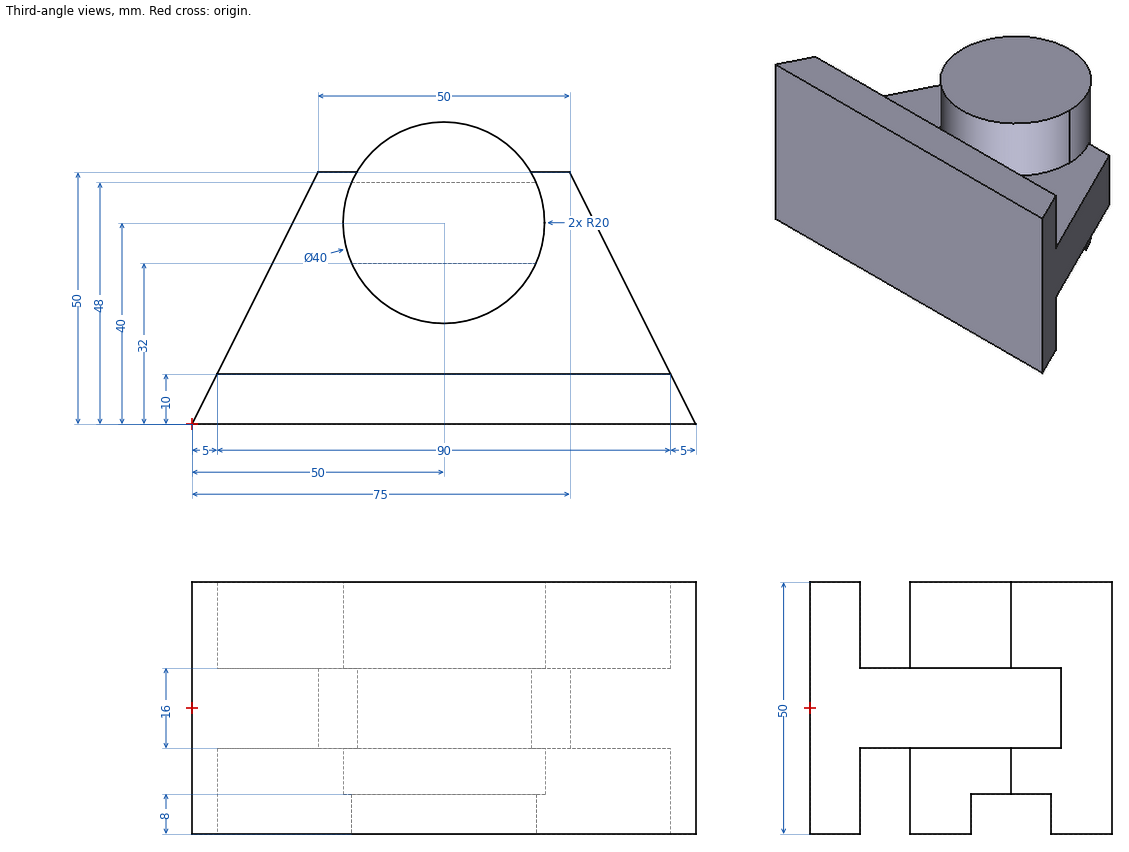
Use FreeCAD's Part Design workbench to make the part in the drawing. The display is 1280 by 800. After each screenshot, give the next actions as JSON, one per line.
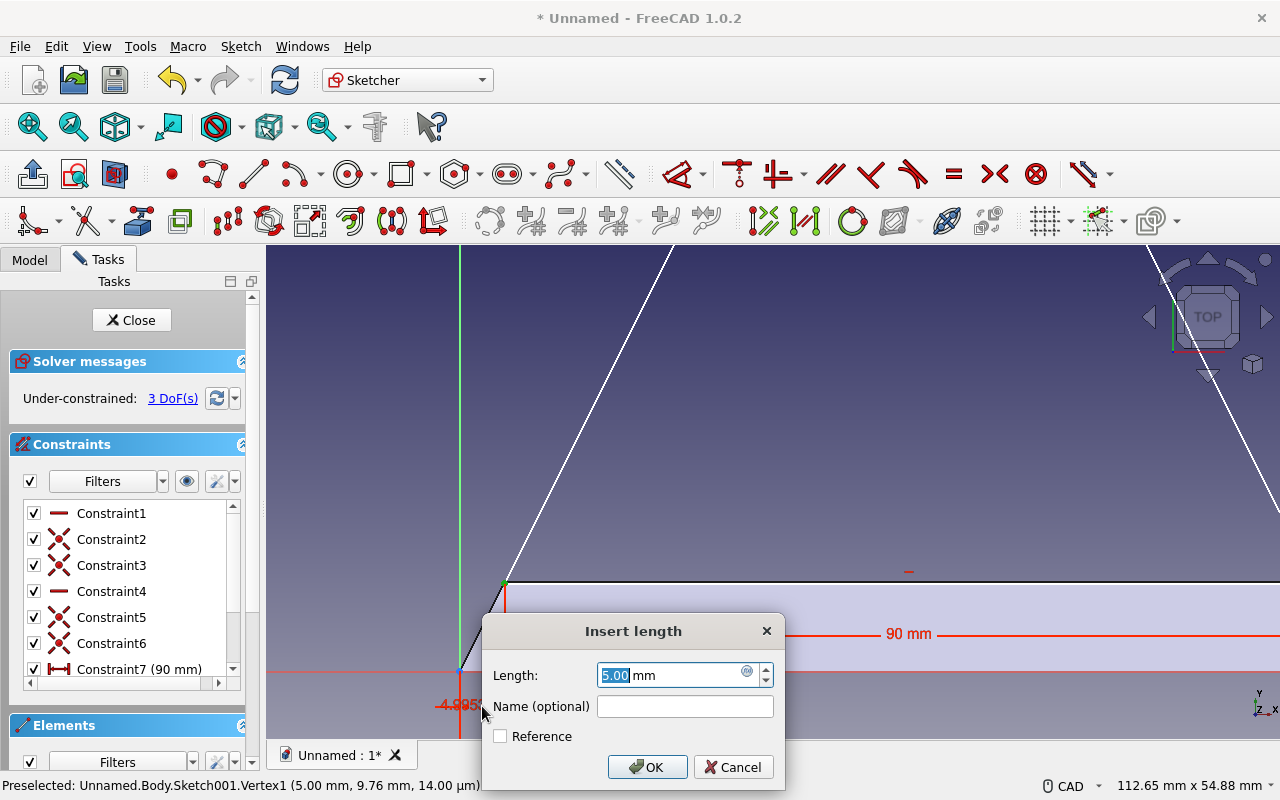
{"action": "type", "text": "5"}
{"action": "key", "text": "Return"}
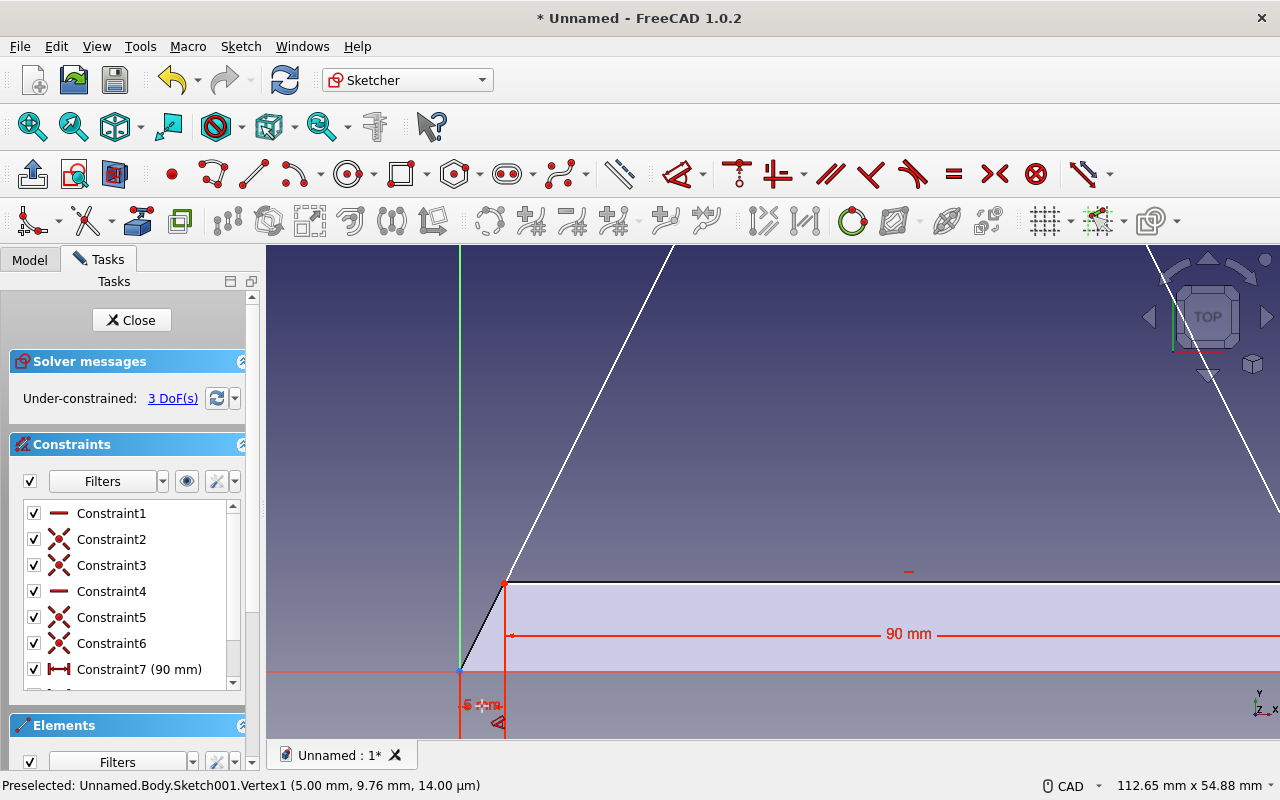
{"action": "left_click", "coordinate": [505, 584]}
{"action": "left_click", "coordinate": [426, 628]}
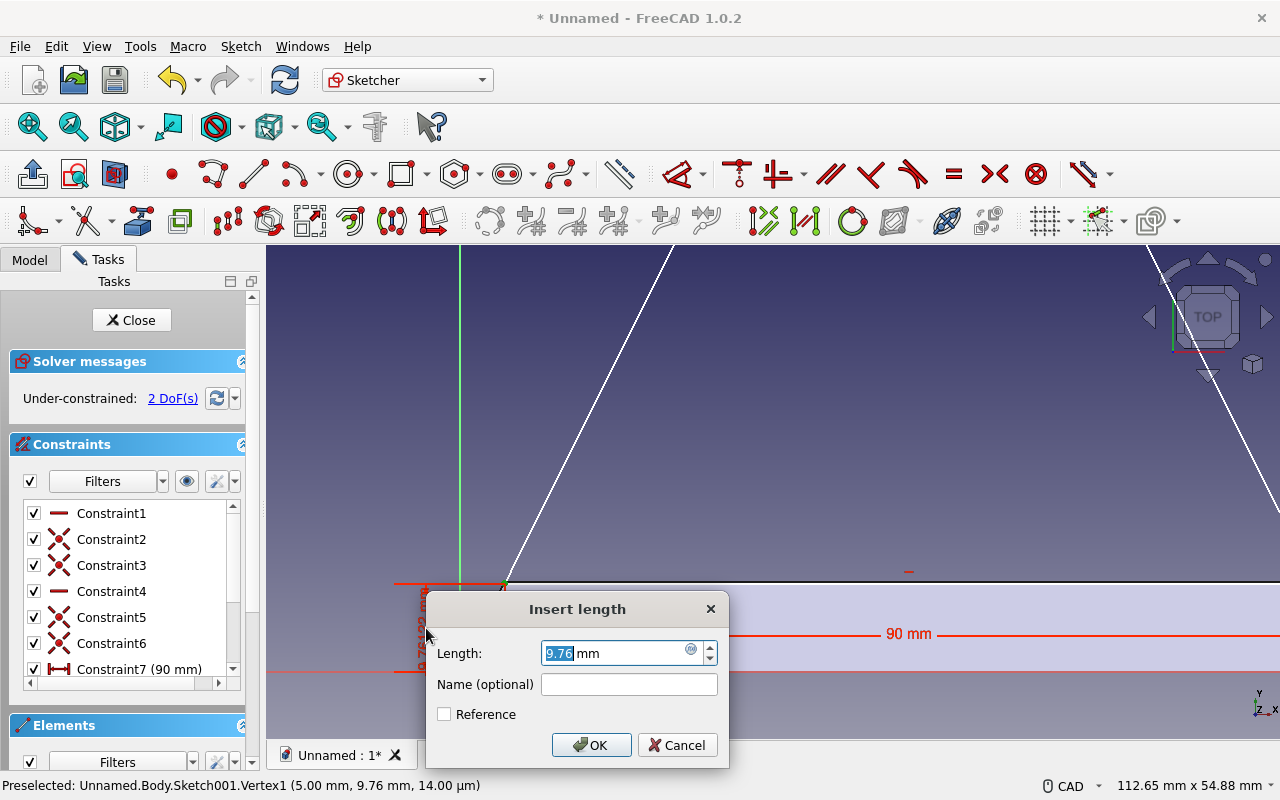
{"action": "type", "text": "10"}
{"action": "key", "text": "Return"}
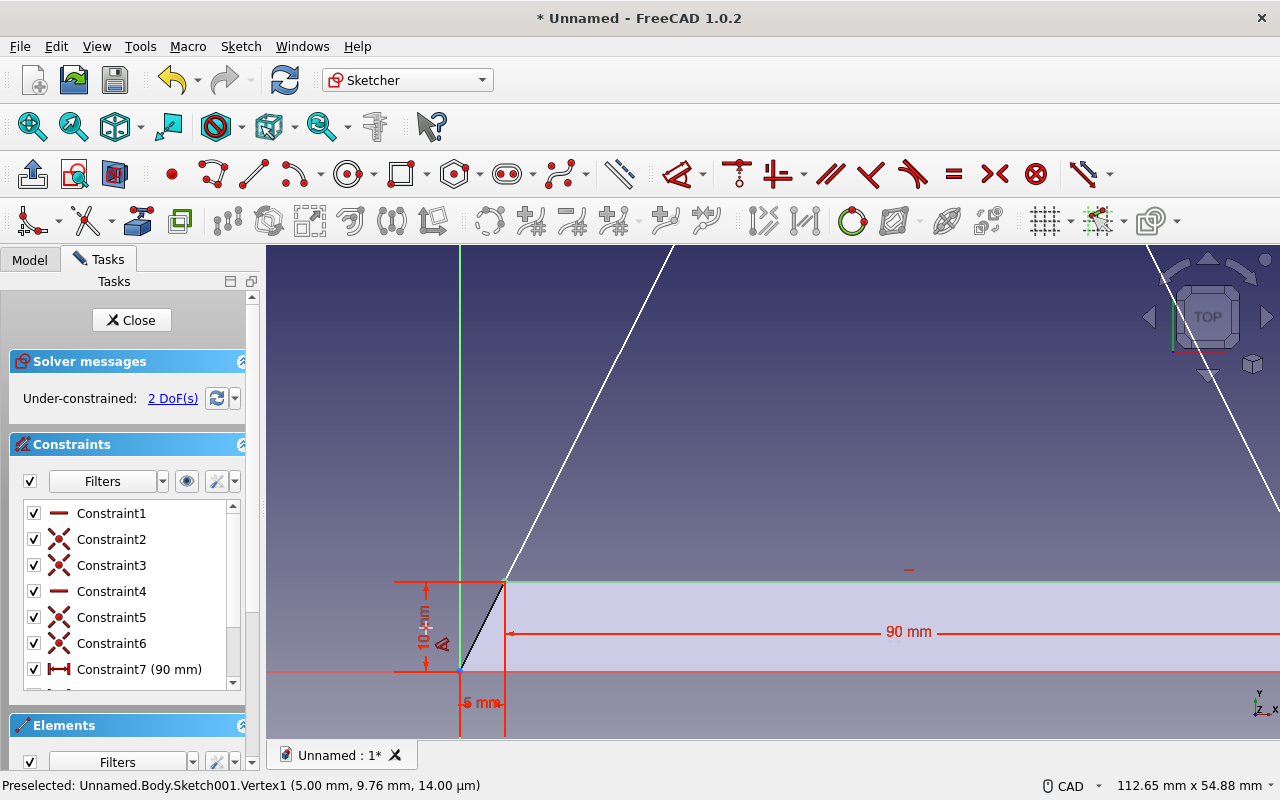
{"action": "scroll", "coordinate": [332, 585], "scroll_direction": "down", "scroll_amount": 2}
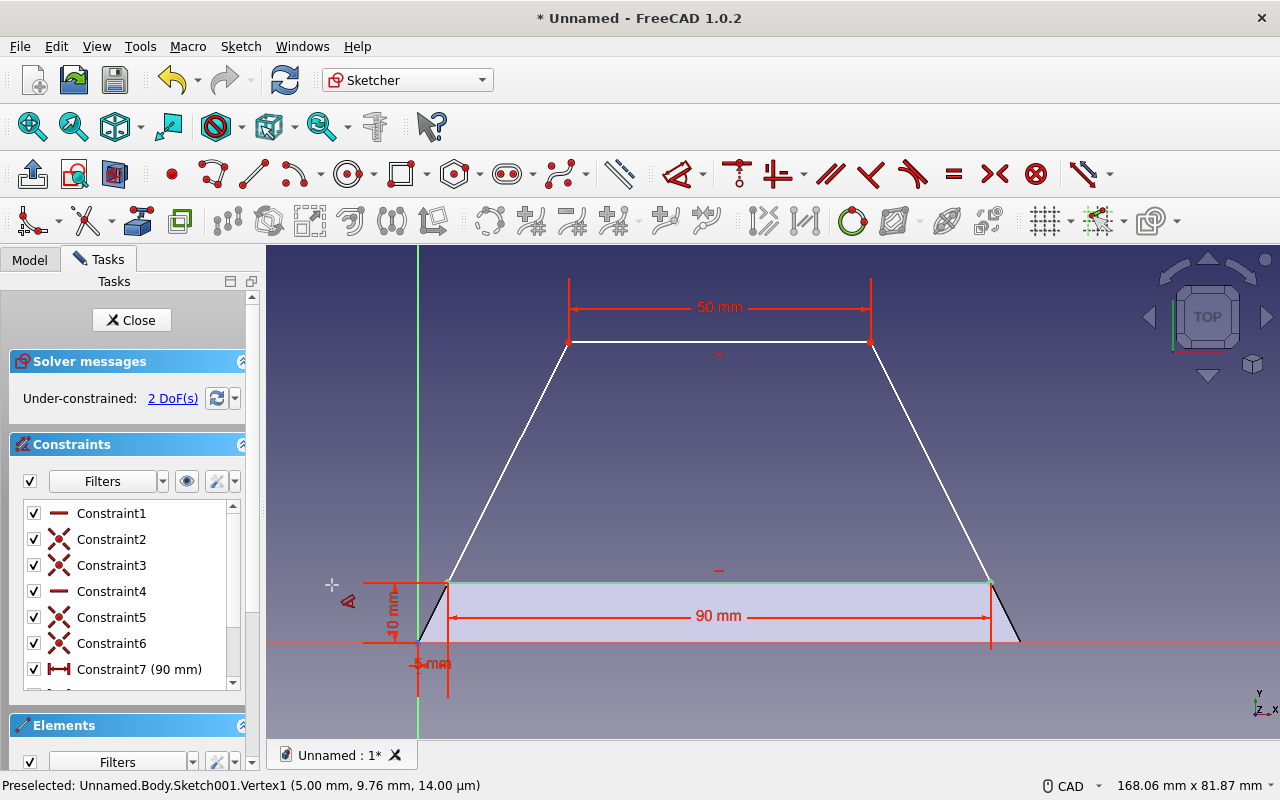
{"action": "left_click", "coordinate": [871, 342]}
{"action": "left_click", "coordinate": [644, 677]}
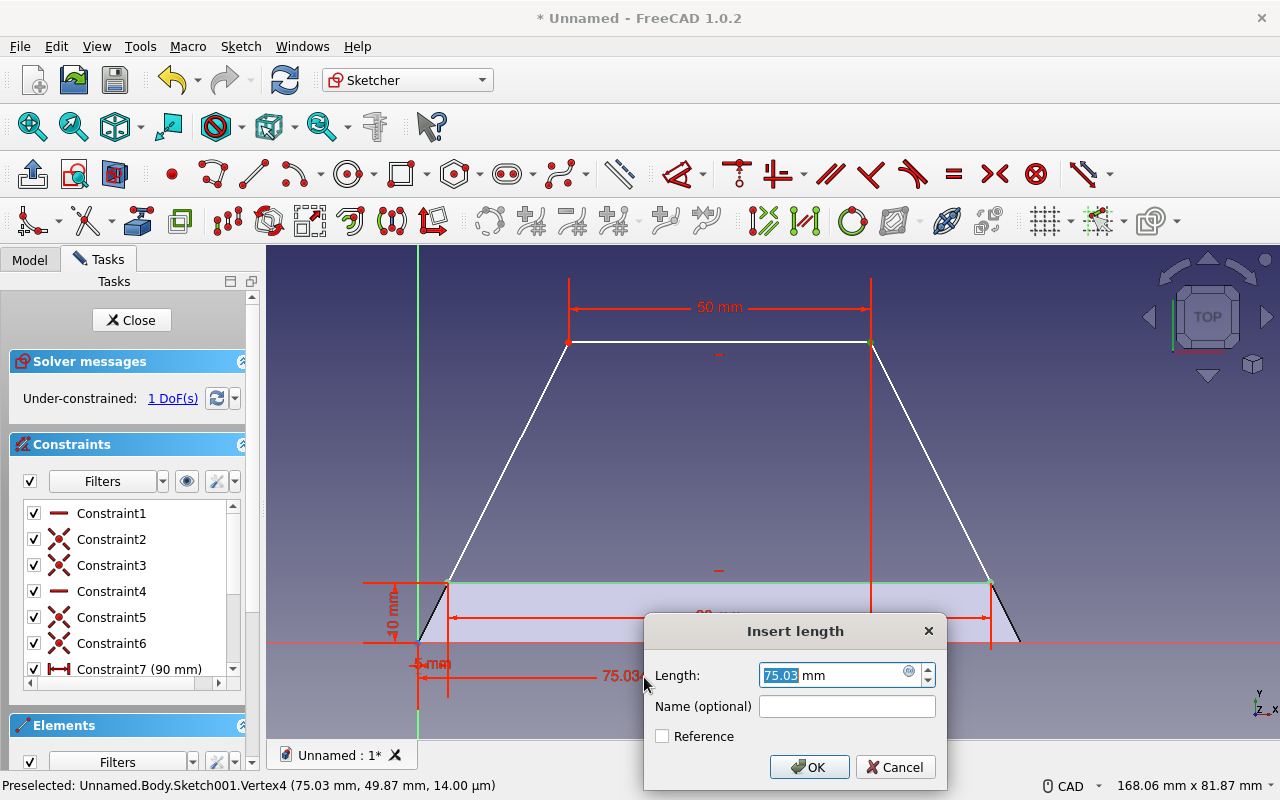
{"action": "type", "text": "75"}
{"action": "key", "text": "Return"}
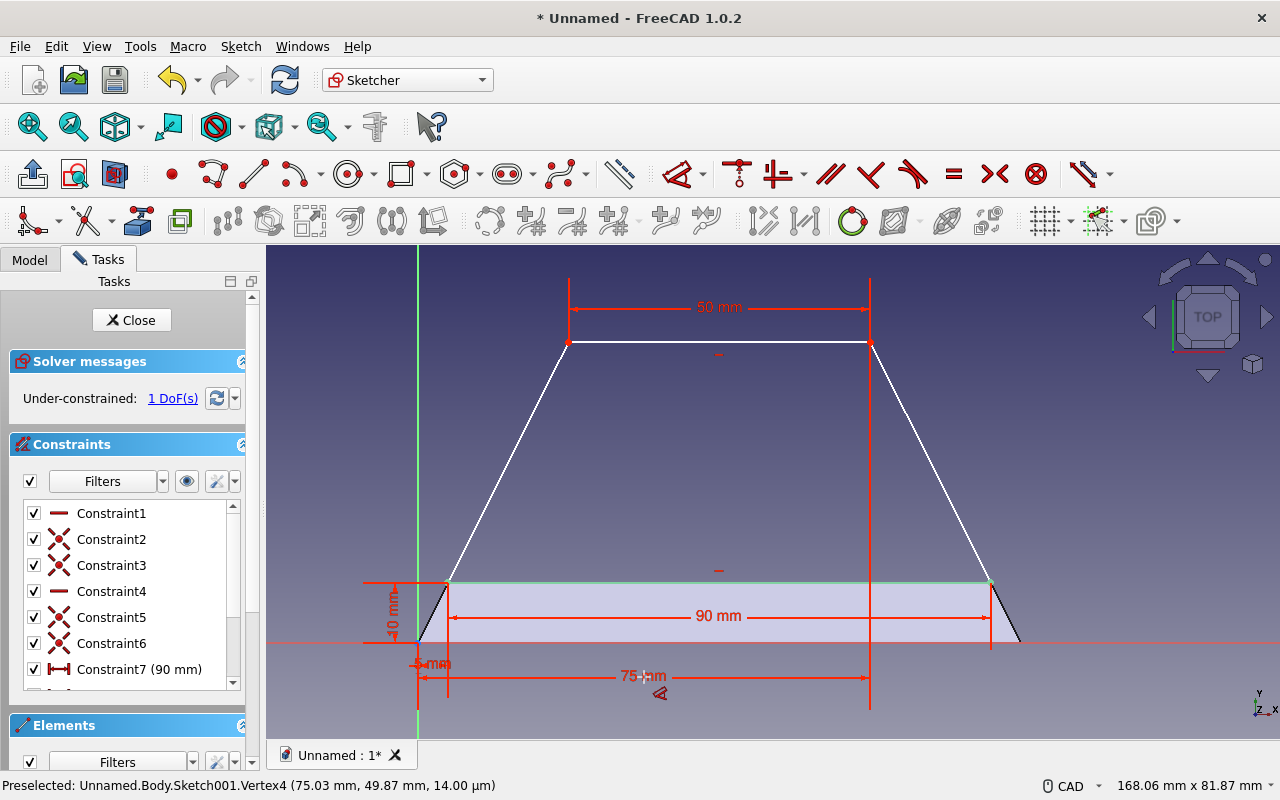
{"action": "left_click", "coordinate": [870, 342]}
{"action": "left_click", "coordinate": [384, 493]}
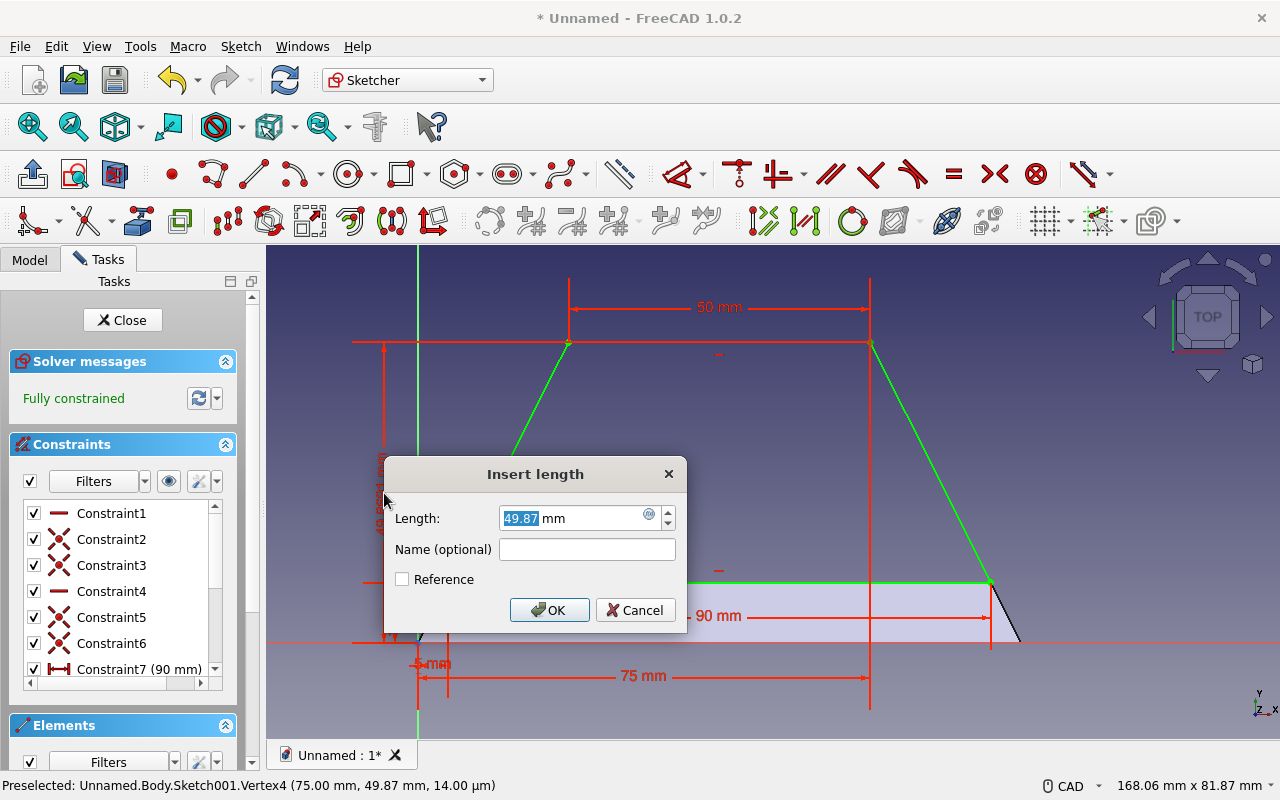
{"action": "type", "text": "50"}
{"action": "key", "text": "Return"}
{"action": "key", "text": "Escape"}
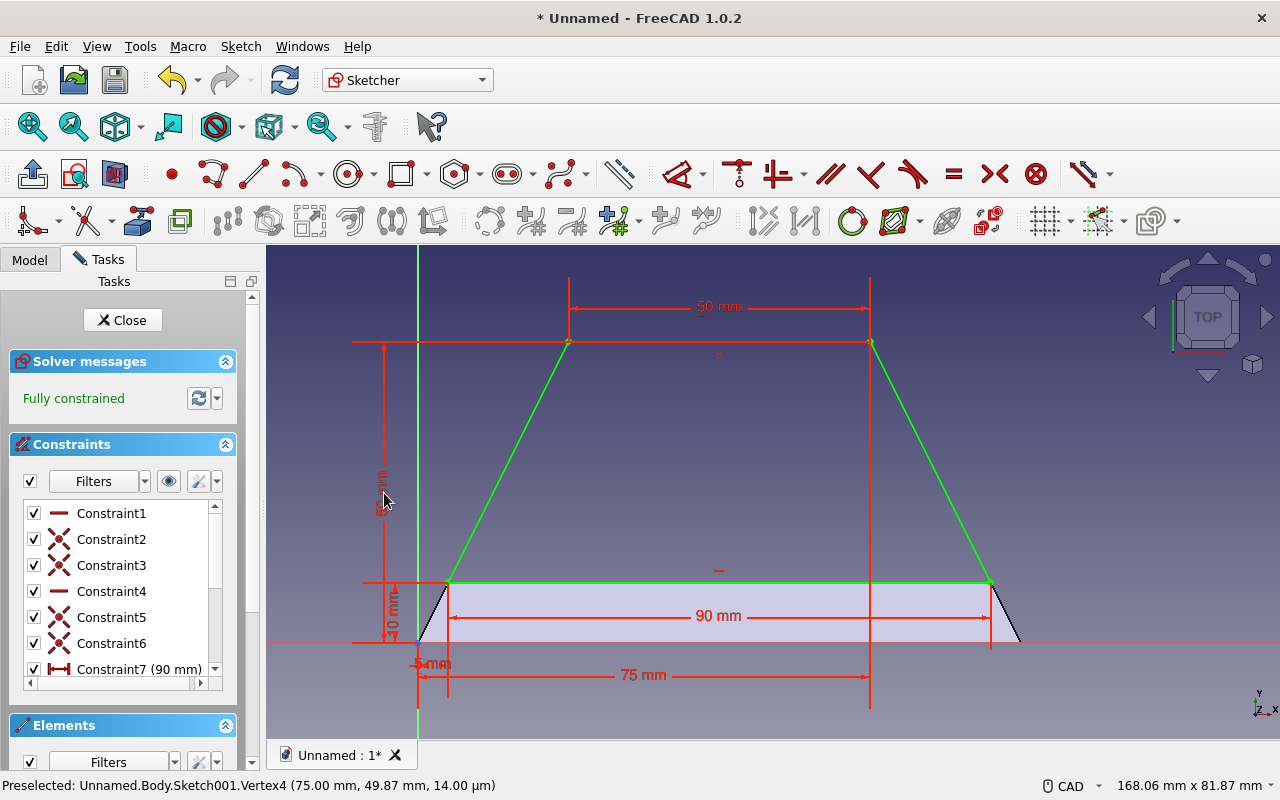
{"action": "left_click", "coordinate": [123, 320]}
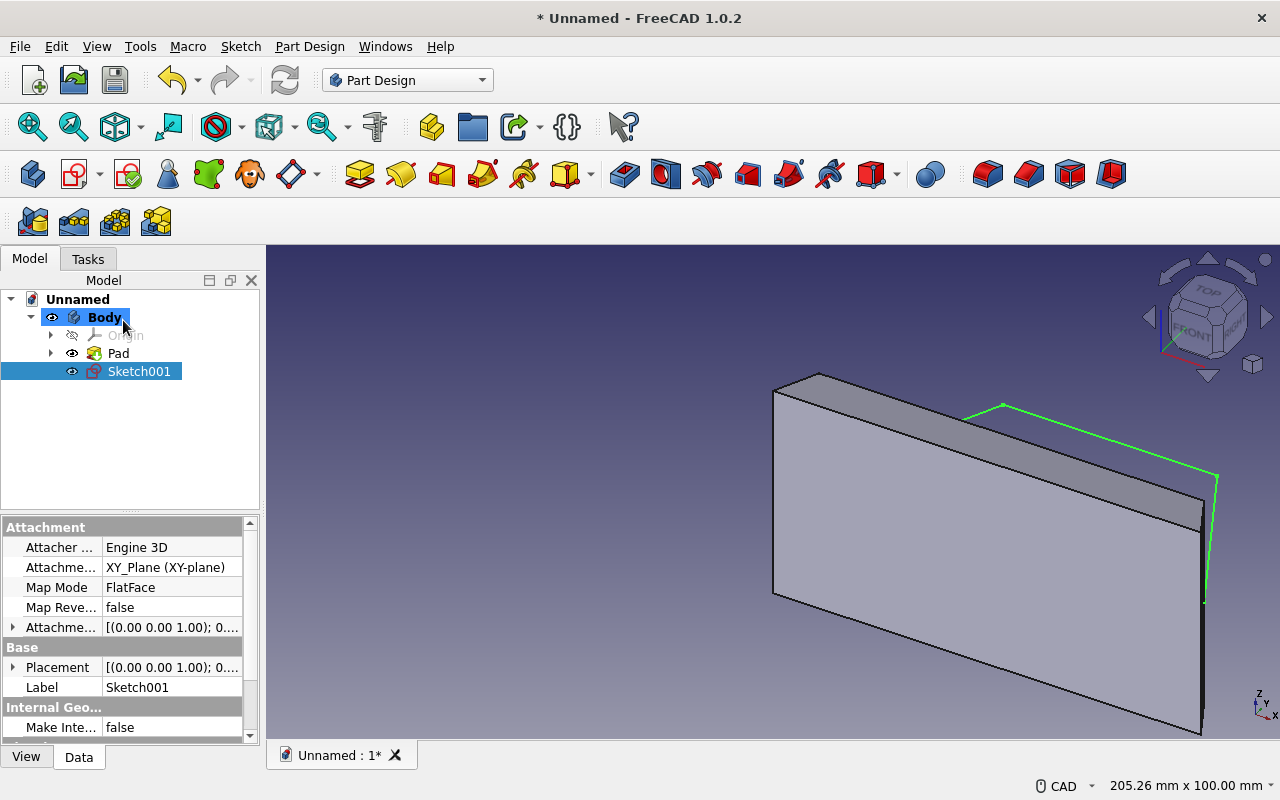
{"action": "left_click", "coordinate": [360, 174]}